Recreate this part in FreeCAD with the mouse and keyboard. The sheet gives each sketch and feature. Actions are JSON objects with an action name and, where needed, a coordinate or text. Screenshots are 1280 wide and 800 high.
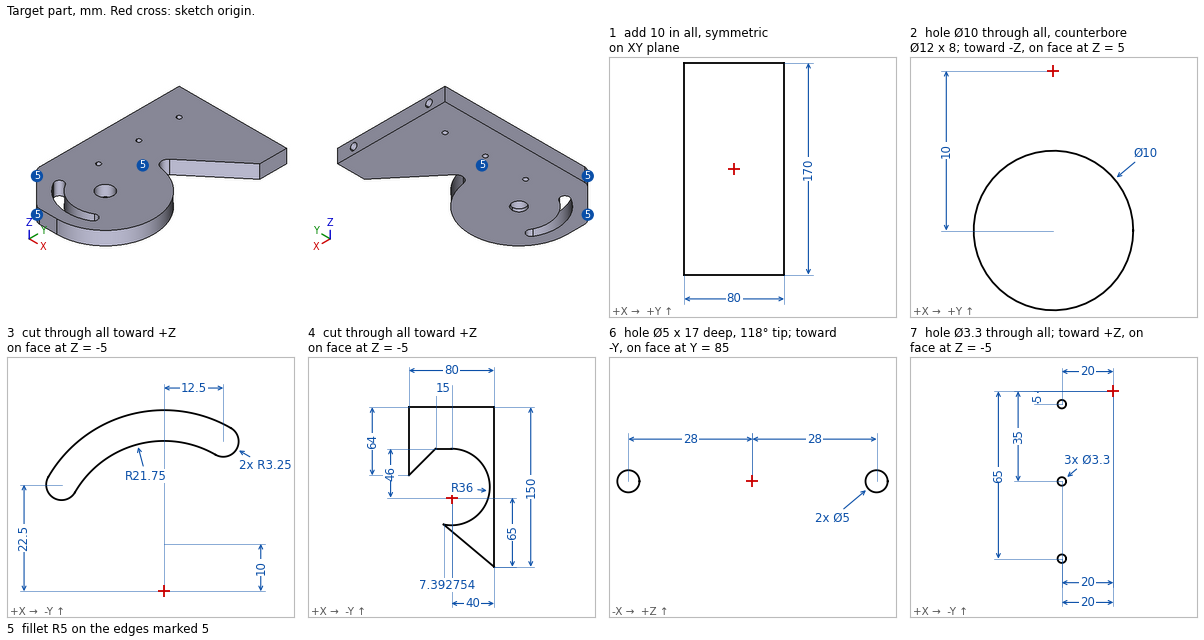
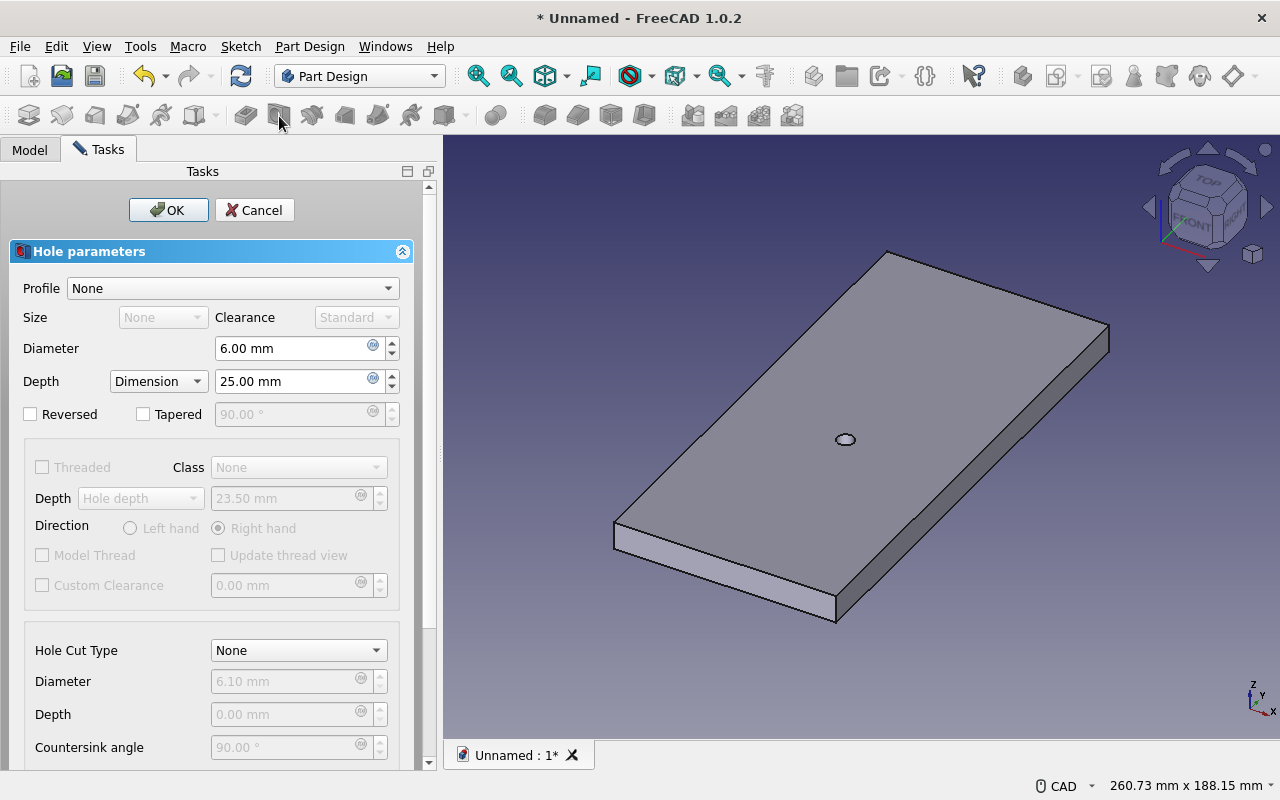
{"action": "triple_click", "coordinate": [300, 348]}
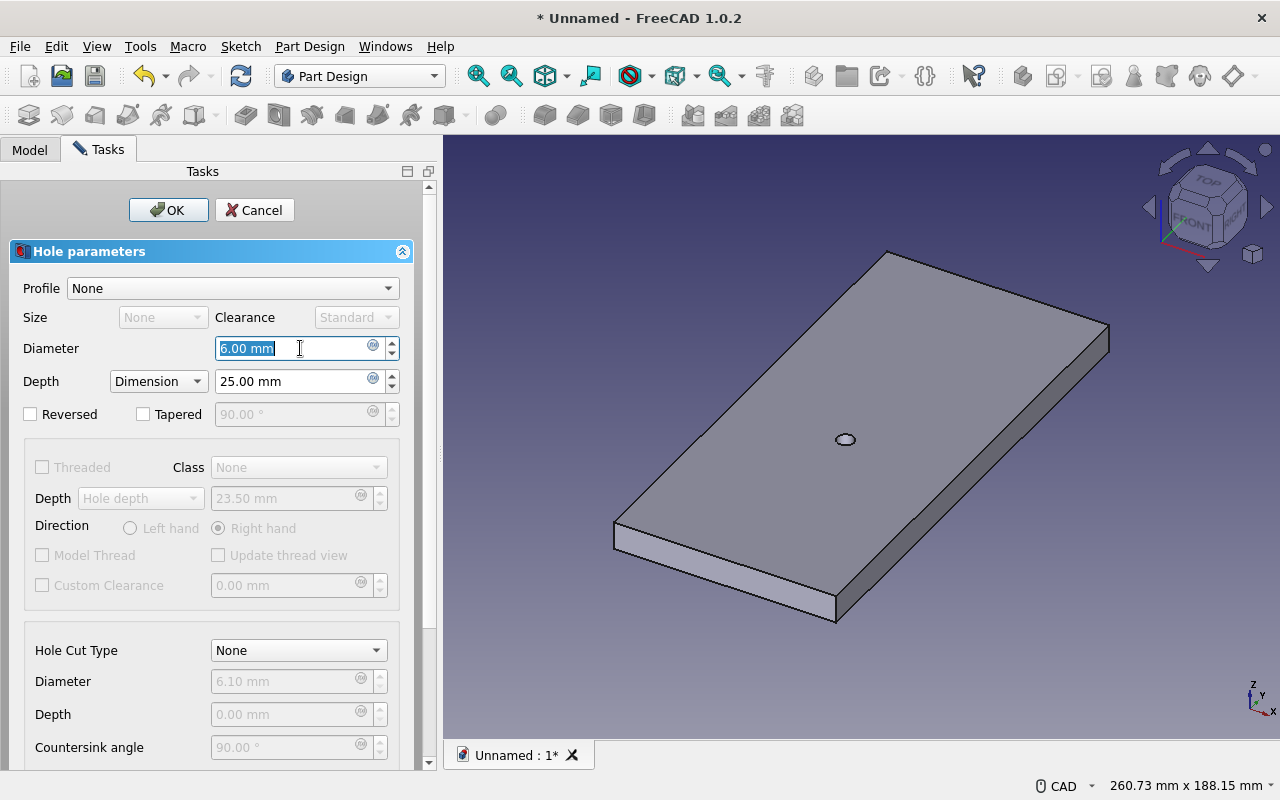
{"action": "type", "text": "10"}
{"action": "key", "text": "Tab"}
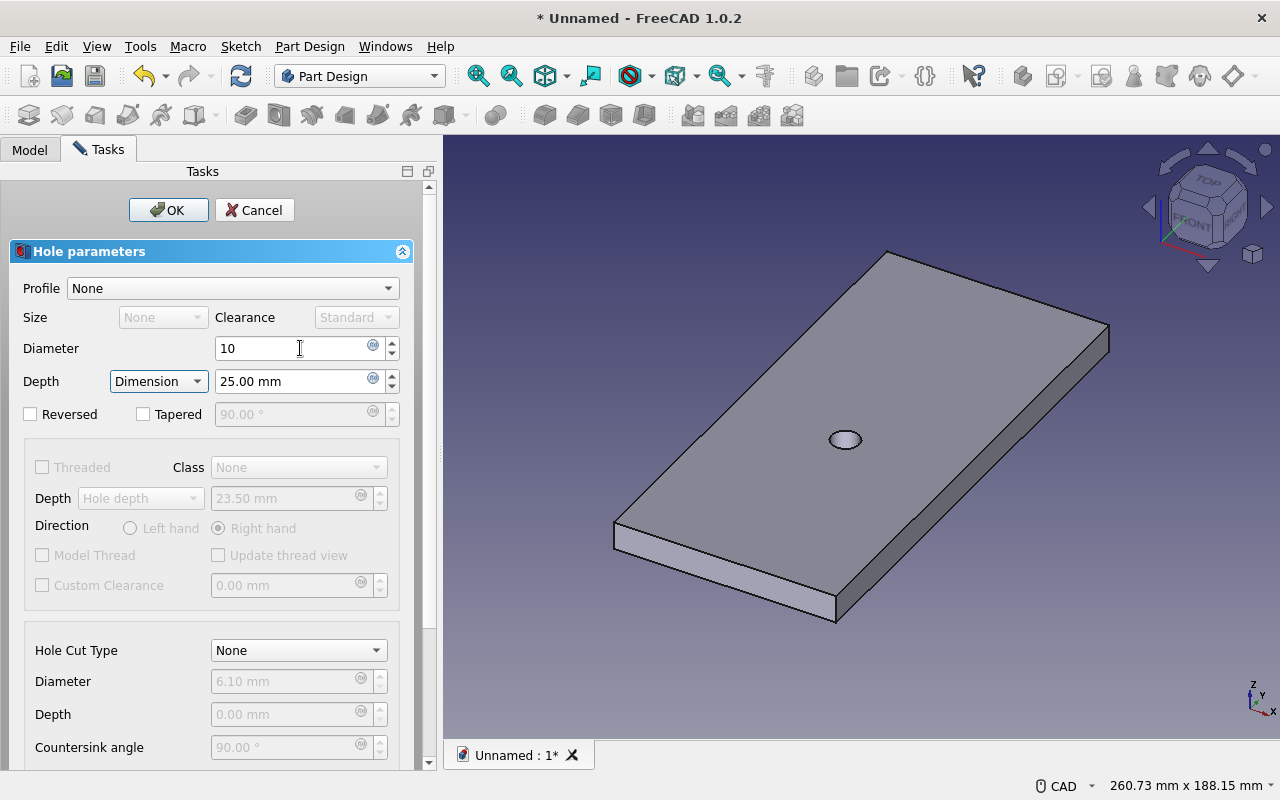
{"action": "left_click", "coordinate": [160, 382]}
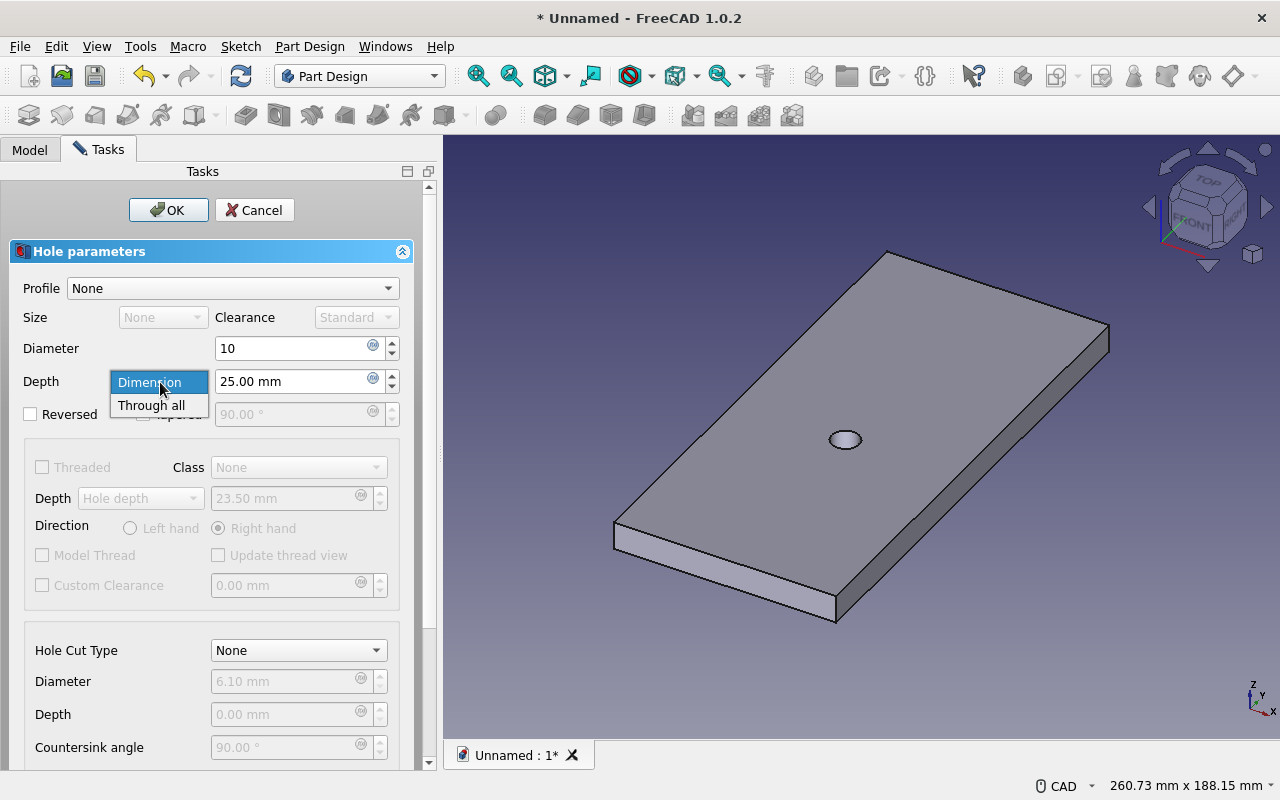
{"action": "left_click", "coordinate": [158, 406]}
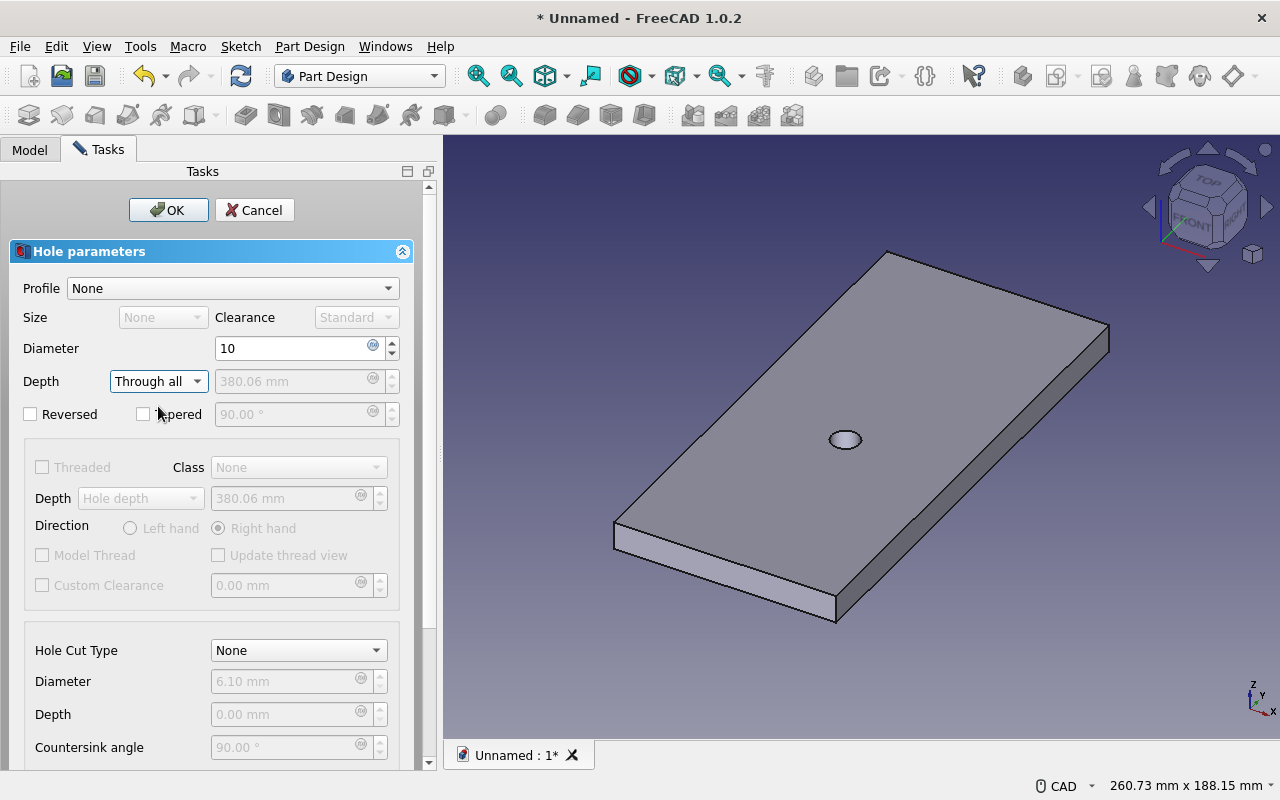
{"action": "left_click", "coordinate": [300, 650]}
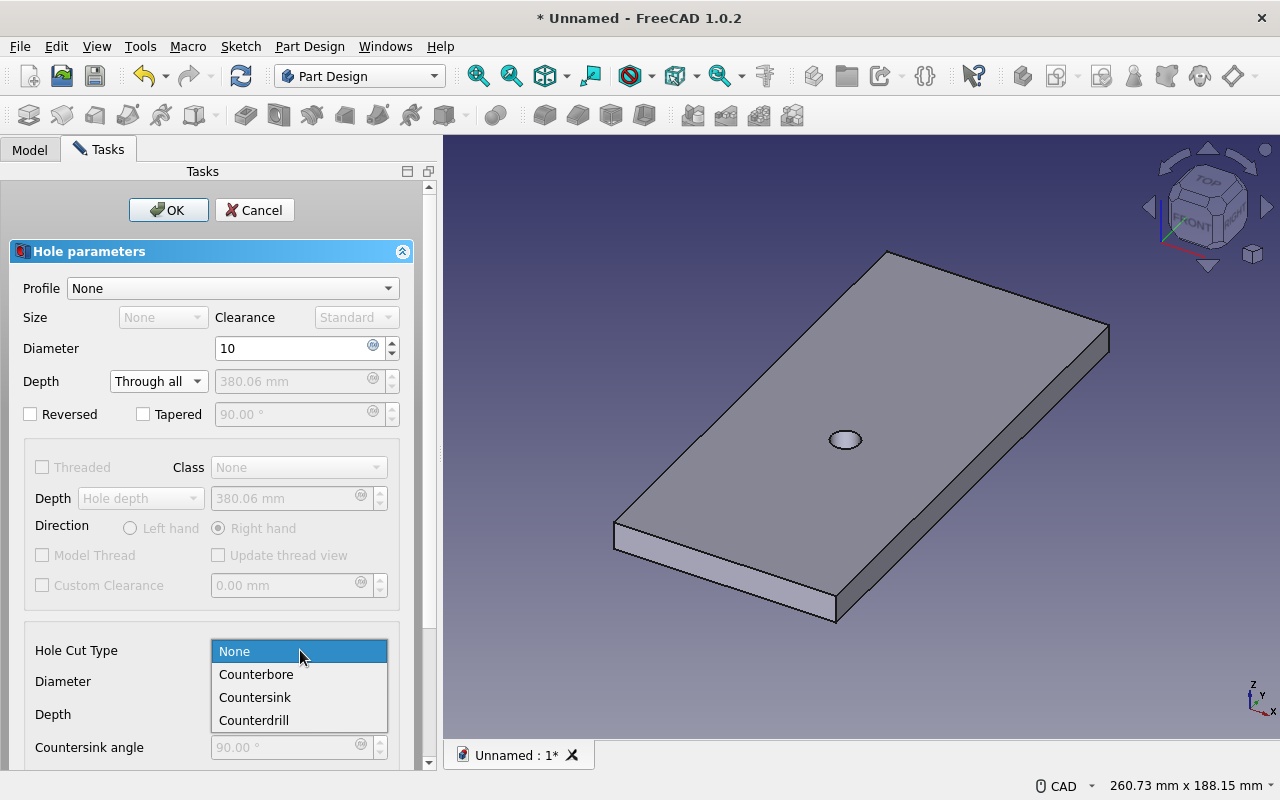
{"action": "left_click", "coordinate": [298, 674]}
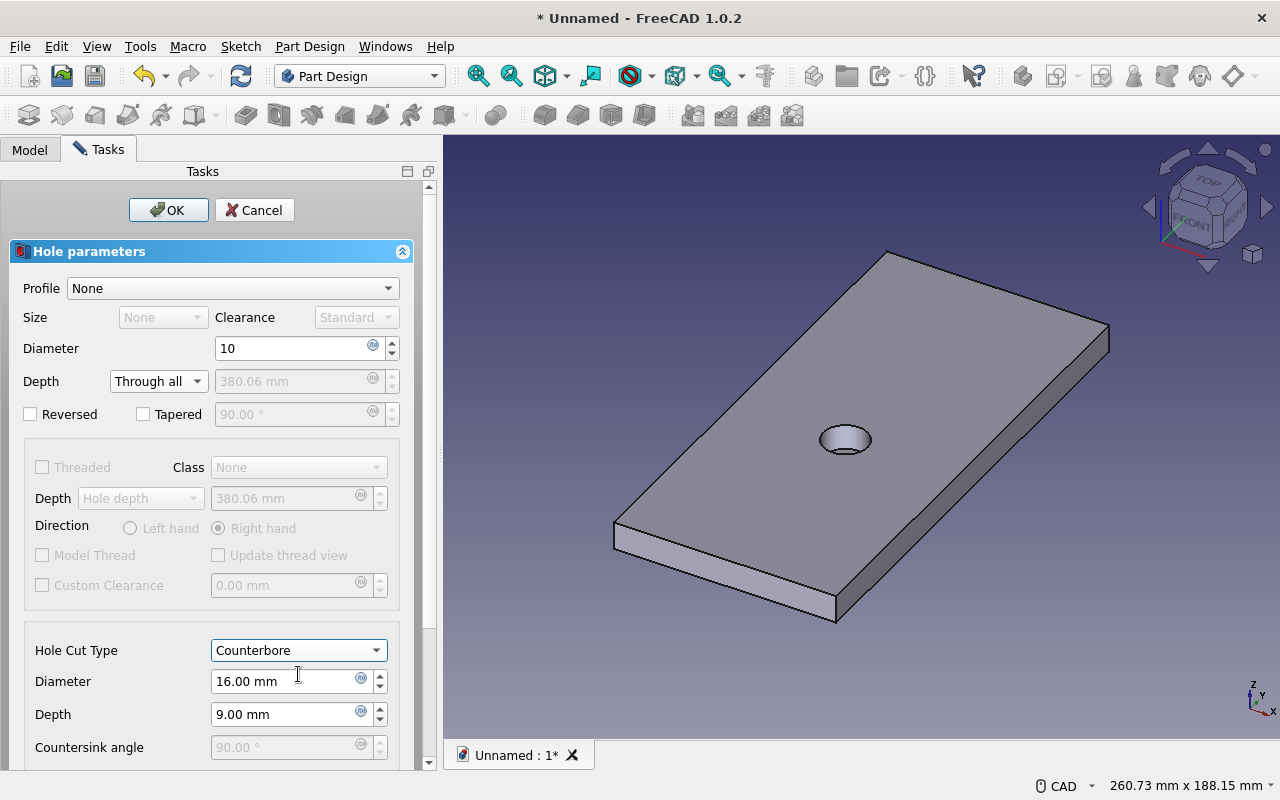
{"action": "triple_click", "coordinate": [292, 682]}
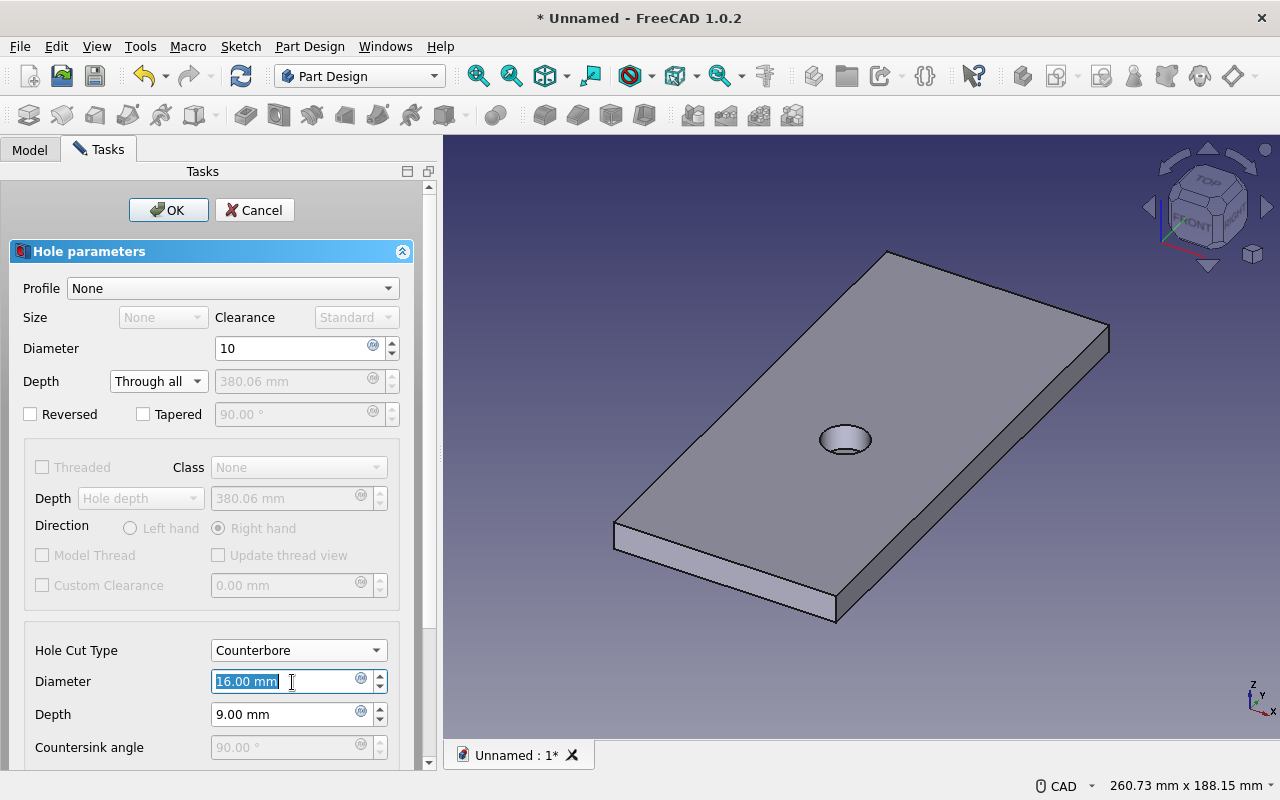
{"action": "type", "text": "12"}
{"action": "key", "text": "Tab"}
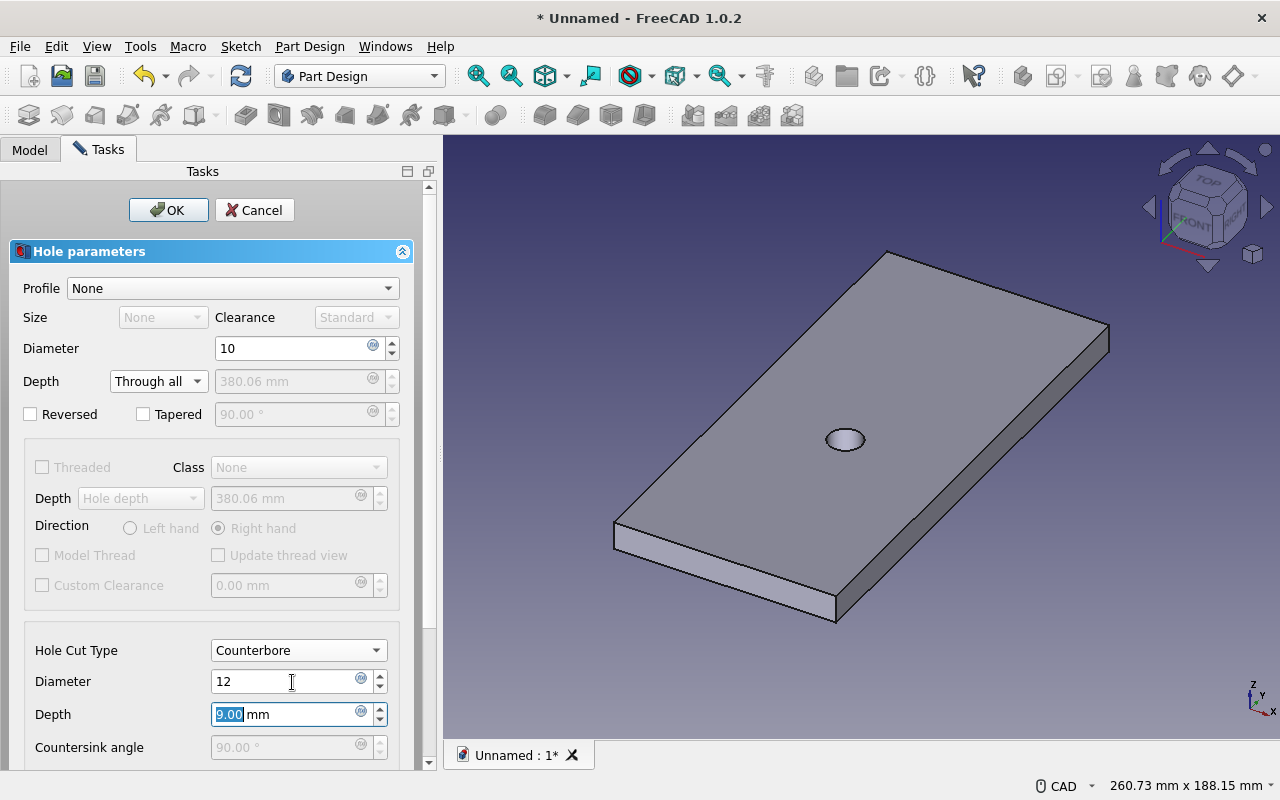
{"action": "type", "text": "8"}
{"action": "key", "text": "Tab"}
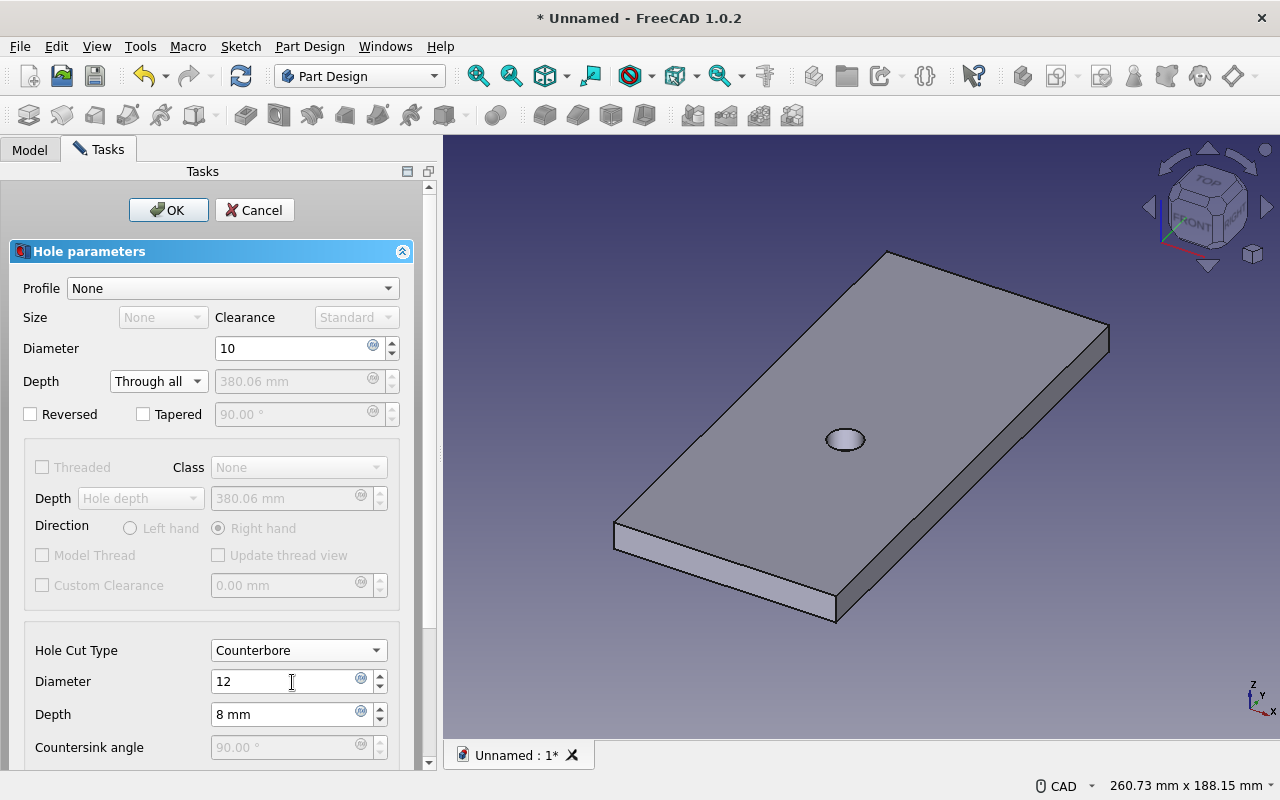
{"action": "left_click", "coordinate": [169, 210]}